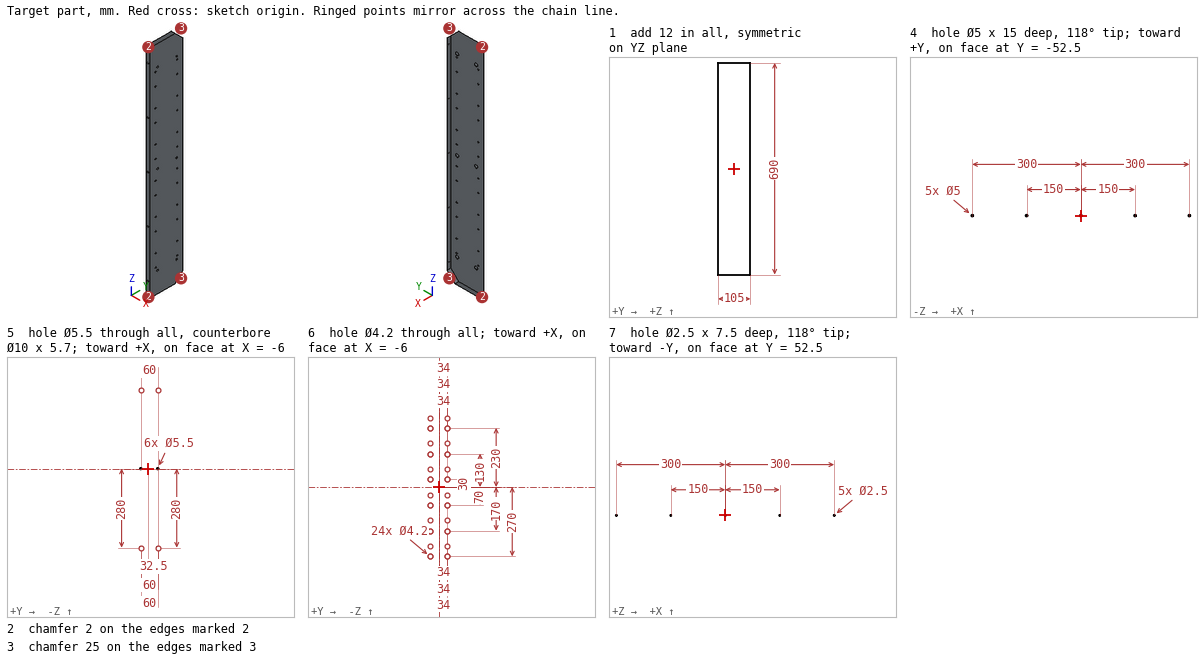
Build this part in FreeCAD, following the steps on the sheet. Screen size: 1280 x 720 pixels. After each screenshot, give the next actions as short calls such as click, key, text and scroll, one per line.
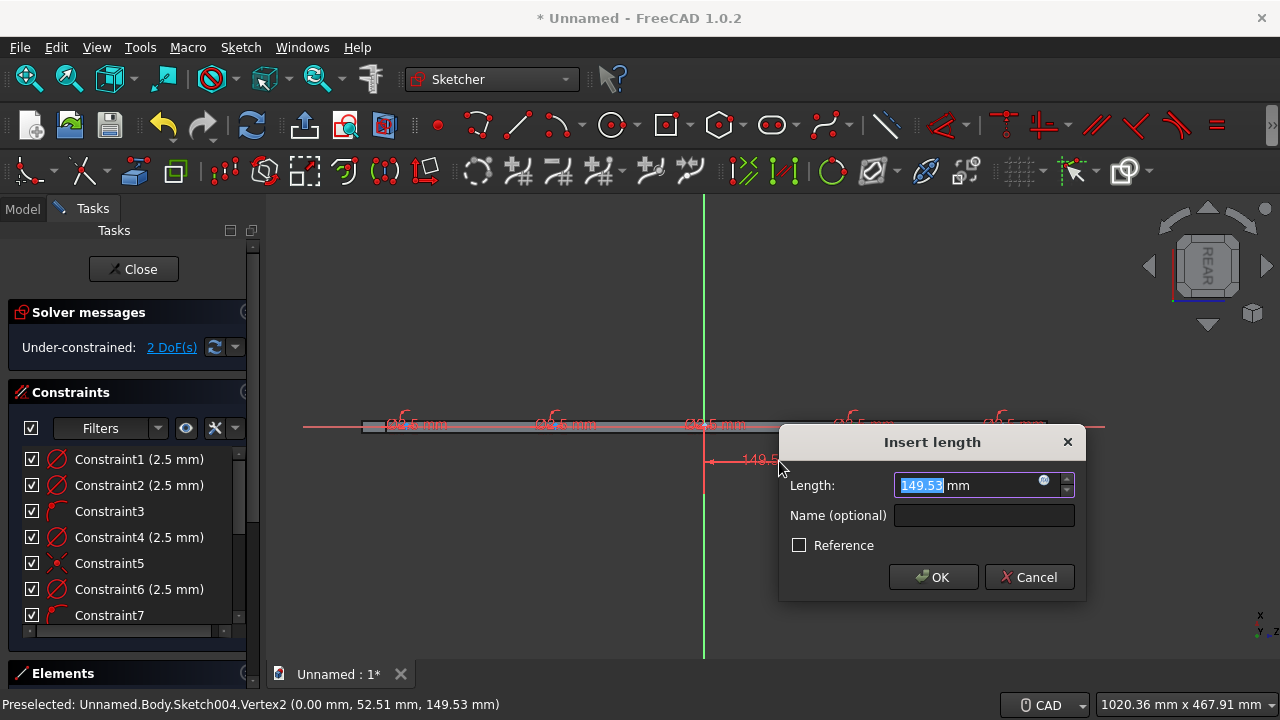
text(150)
key(Return)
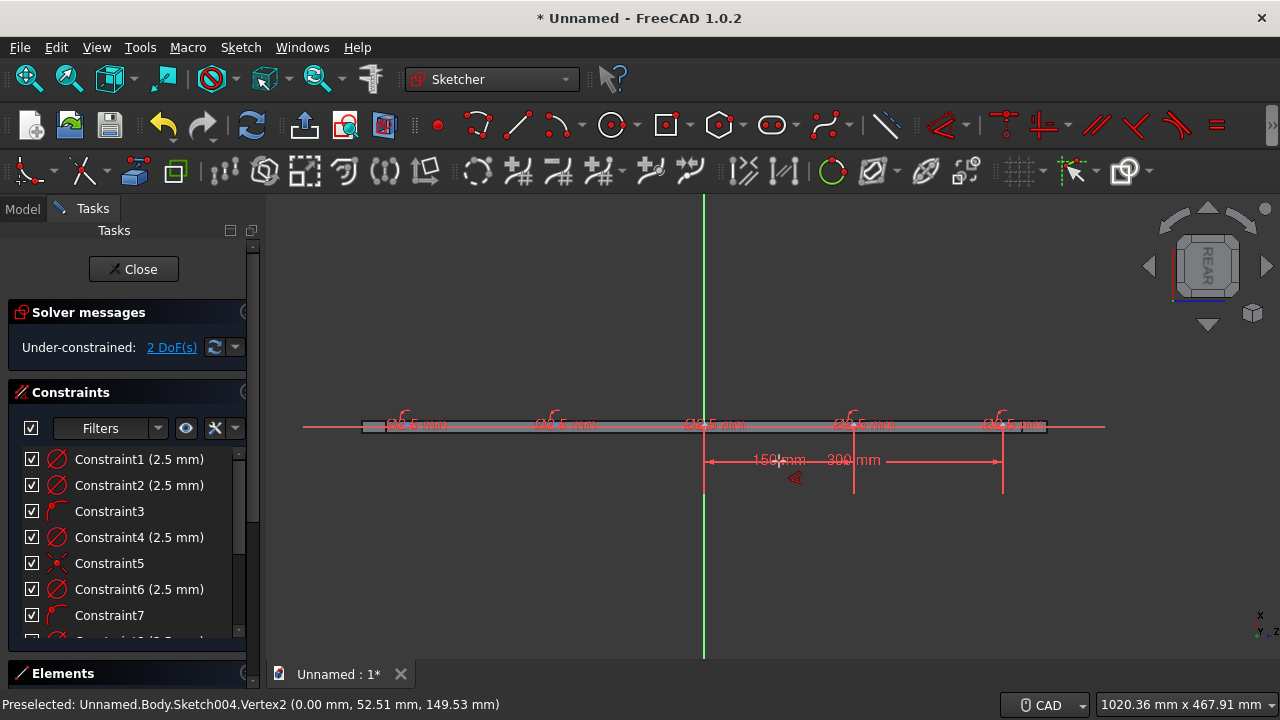
click(555, 427)
click(630, 461)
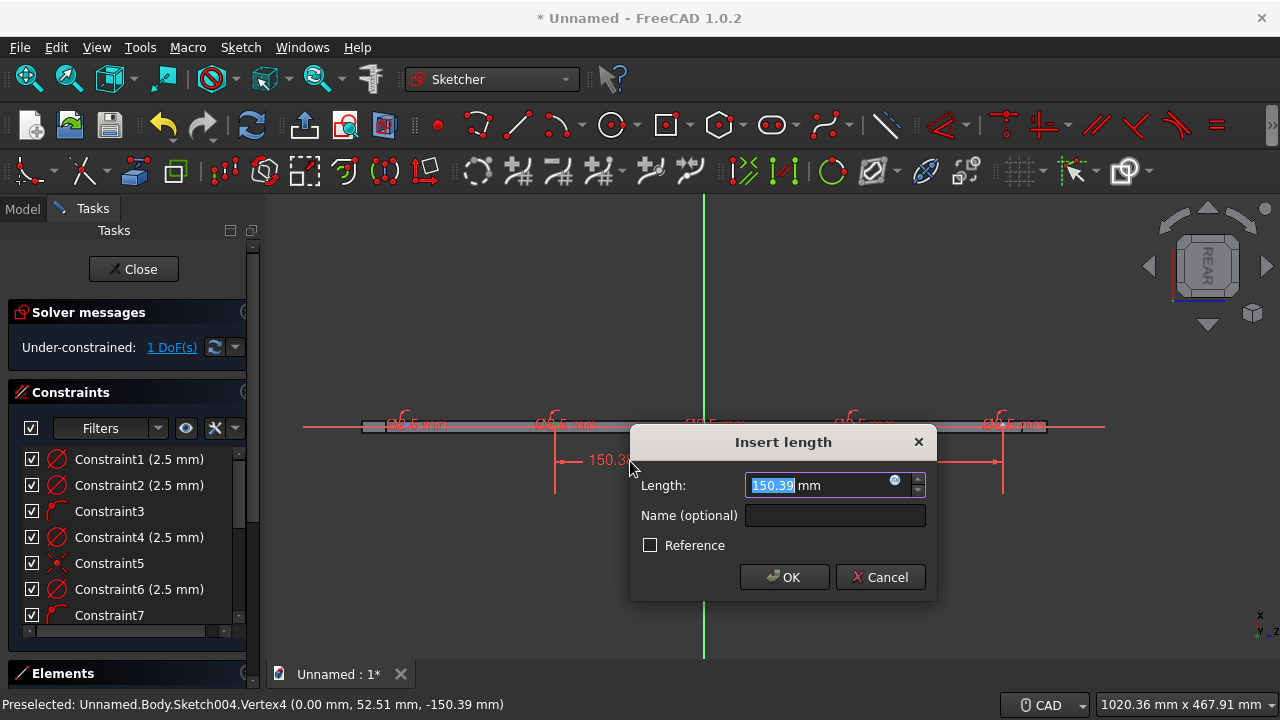
text(150)
key(Return)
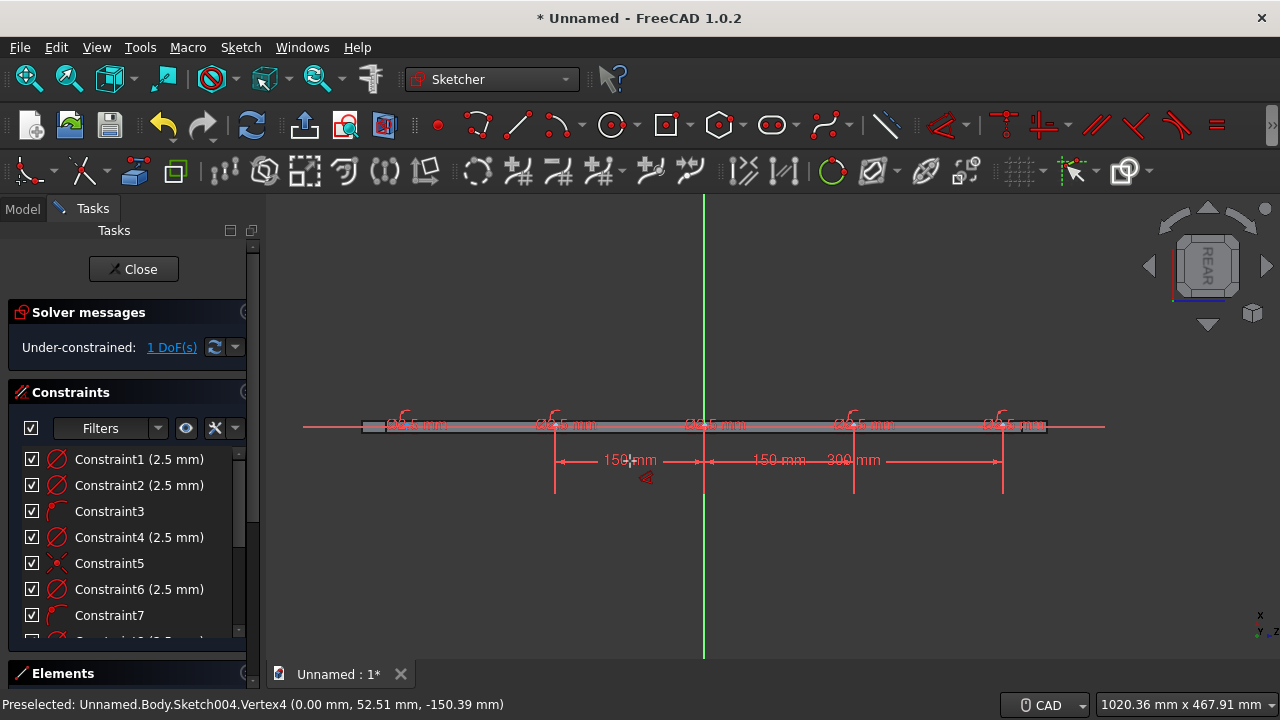
click(406, 427)
click(555, 461)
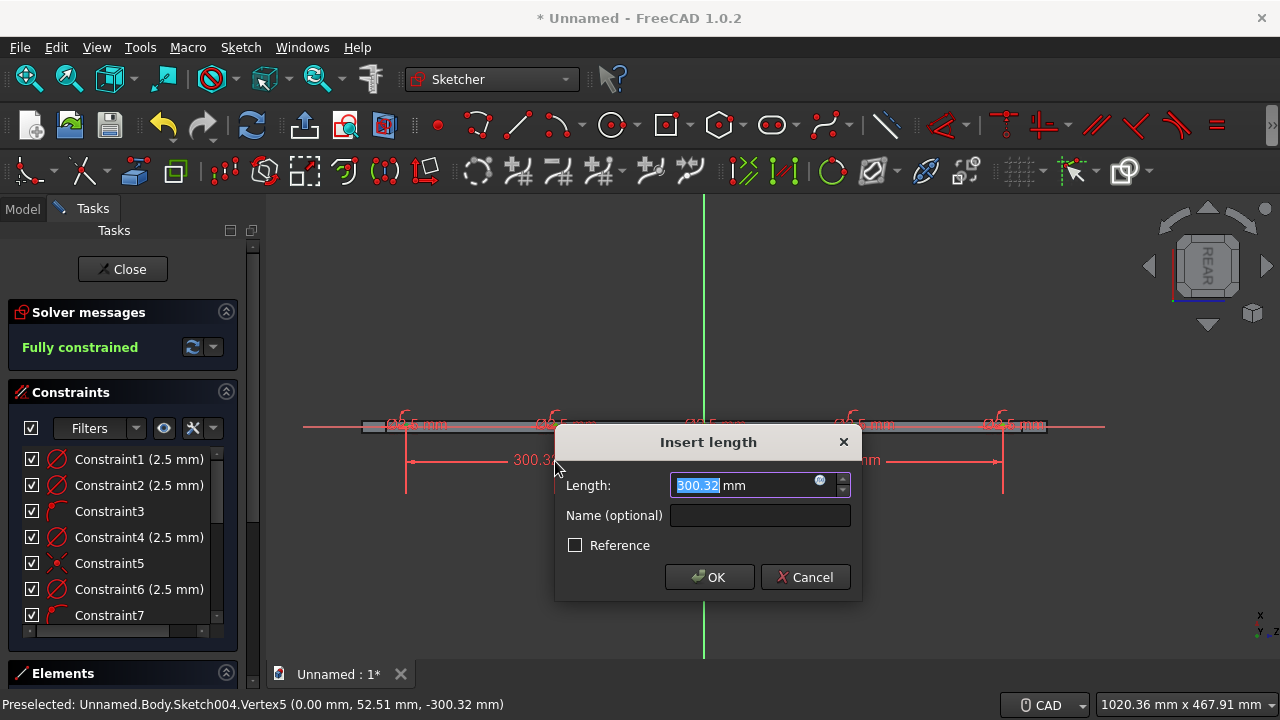
text(300)
key(Return)
key(Escape)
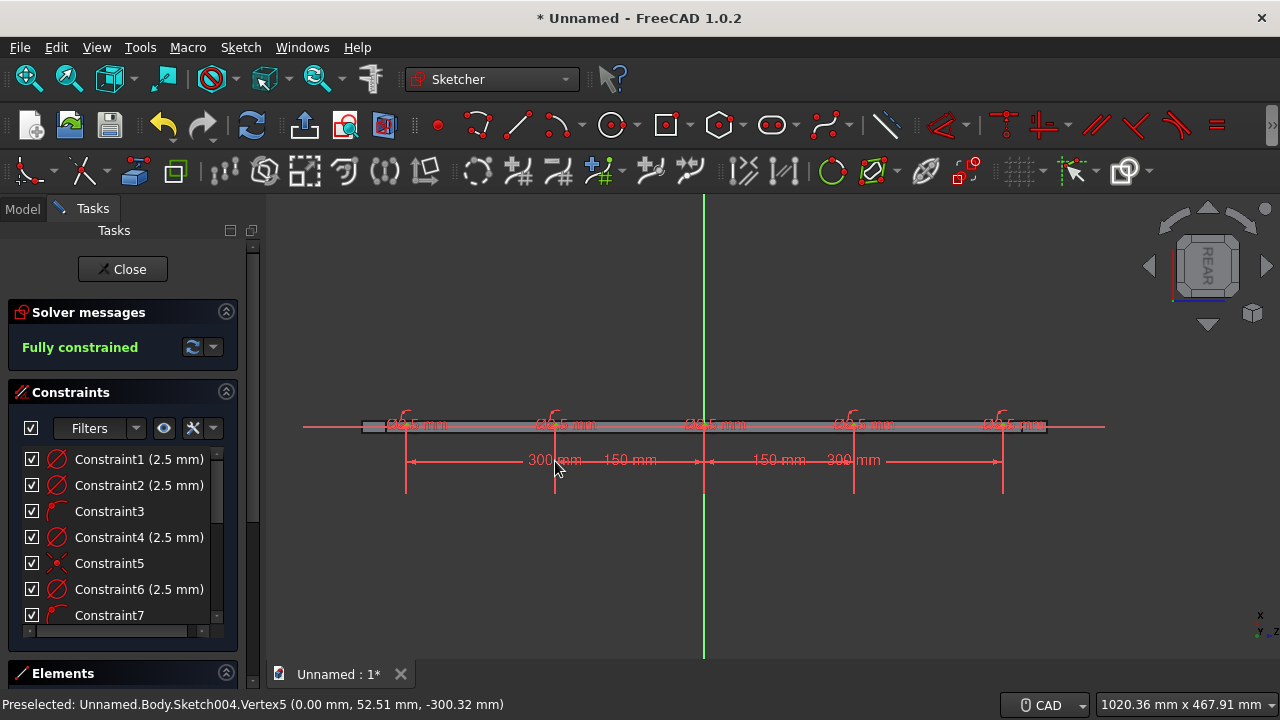
click(123, 269)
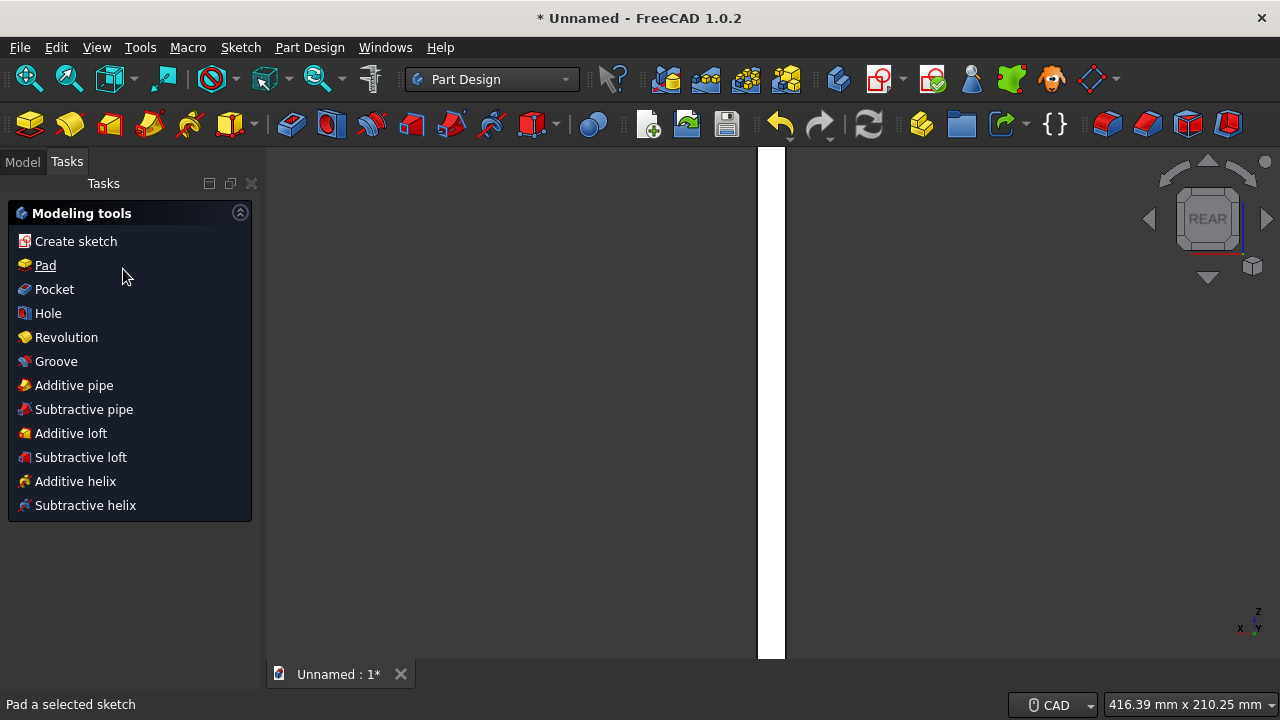
click(332, 124)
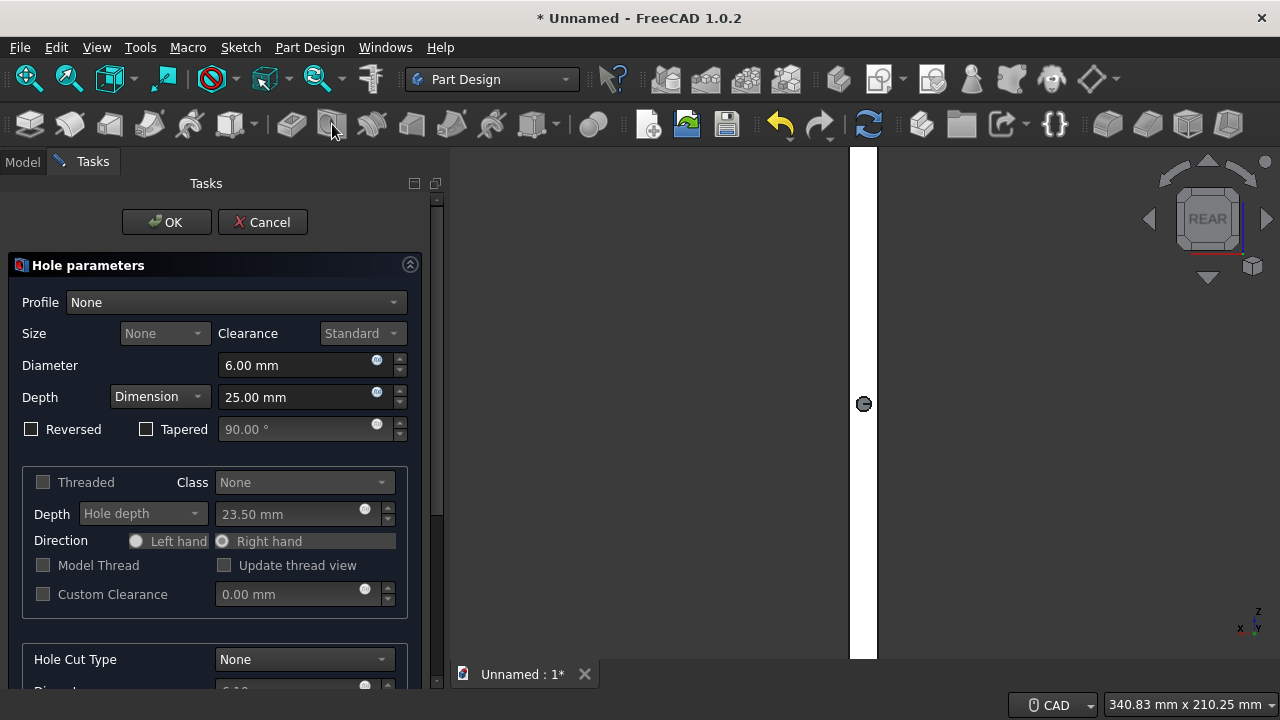
triple_click(305, 365)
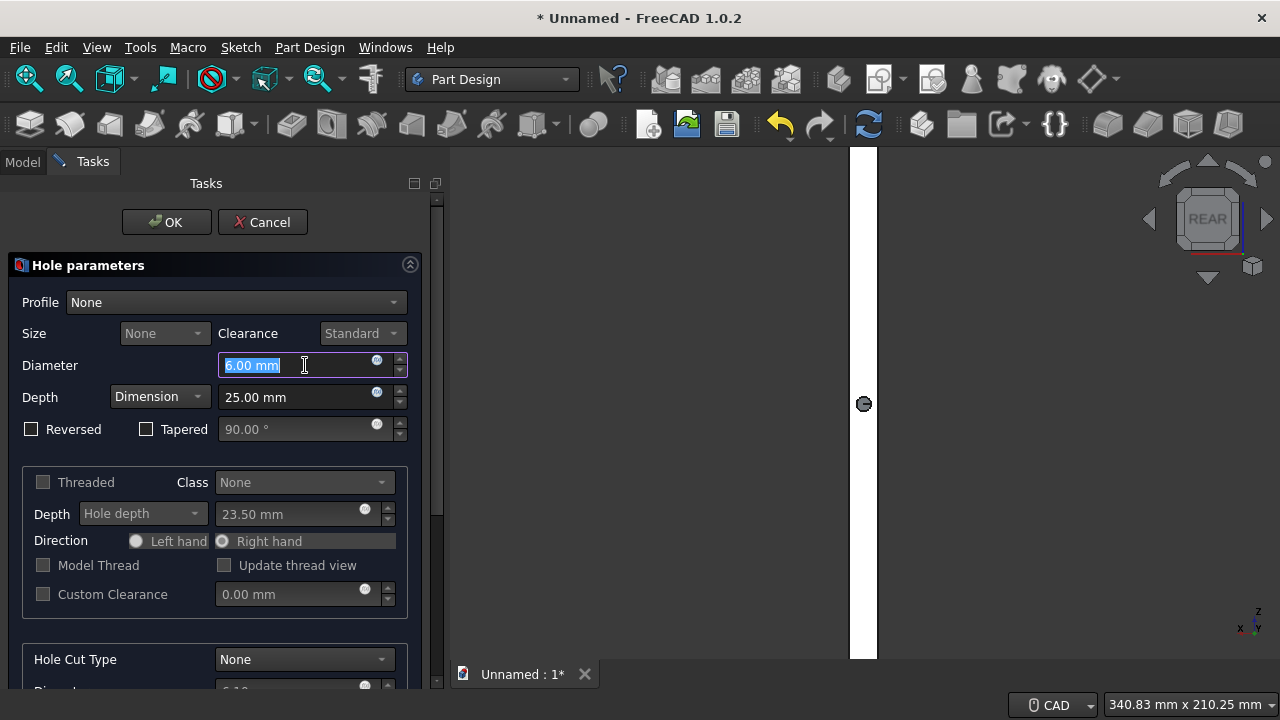
text(2.5)
key(Tab)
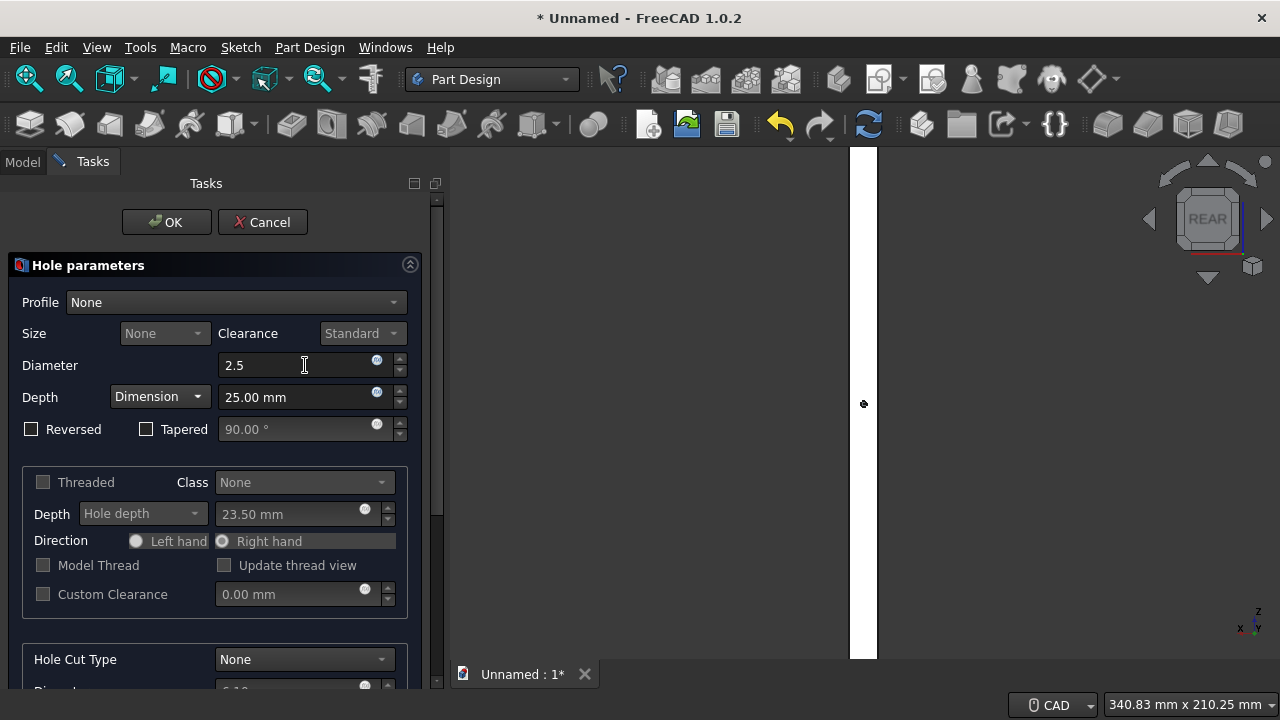
triple_click(305, 397)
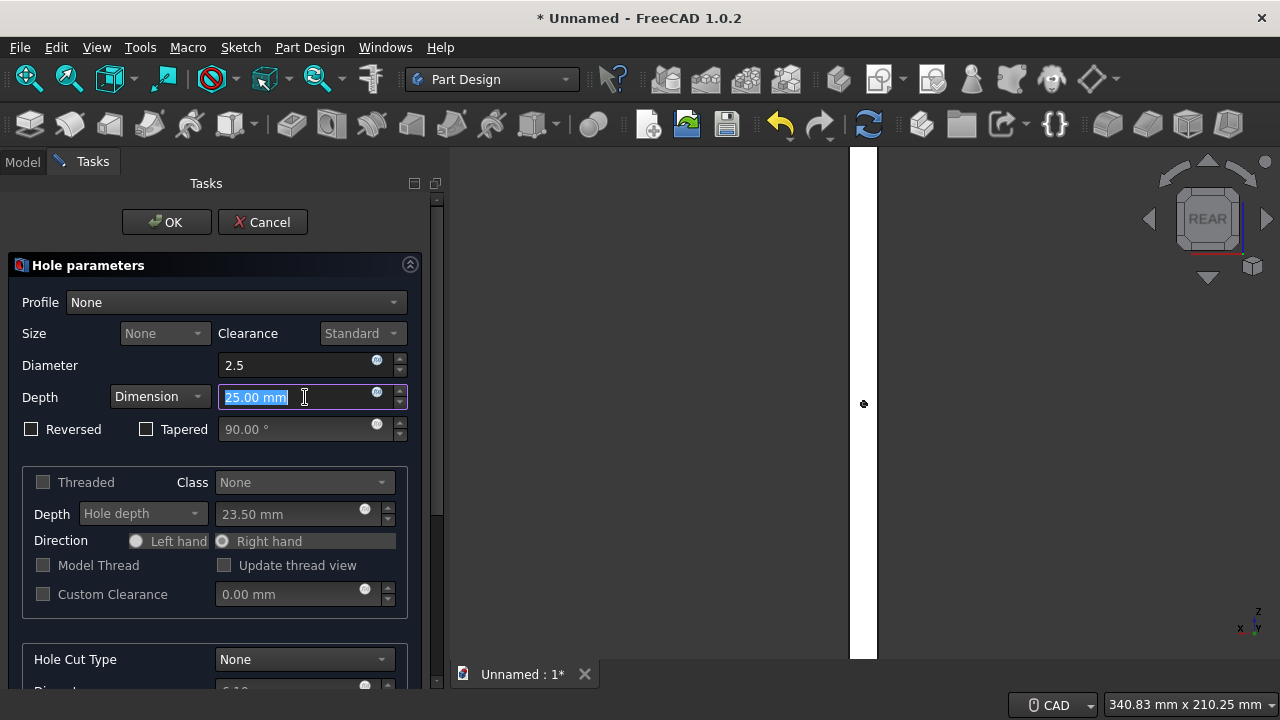
text(7.5)
key(Tab)